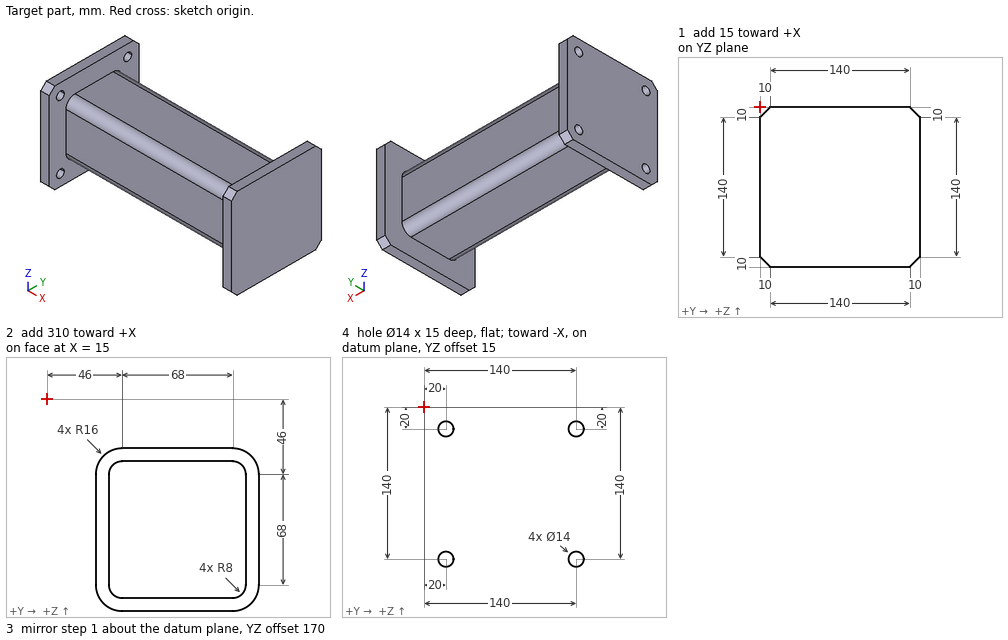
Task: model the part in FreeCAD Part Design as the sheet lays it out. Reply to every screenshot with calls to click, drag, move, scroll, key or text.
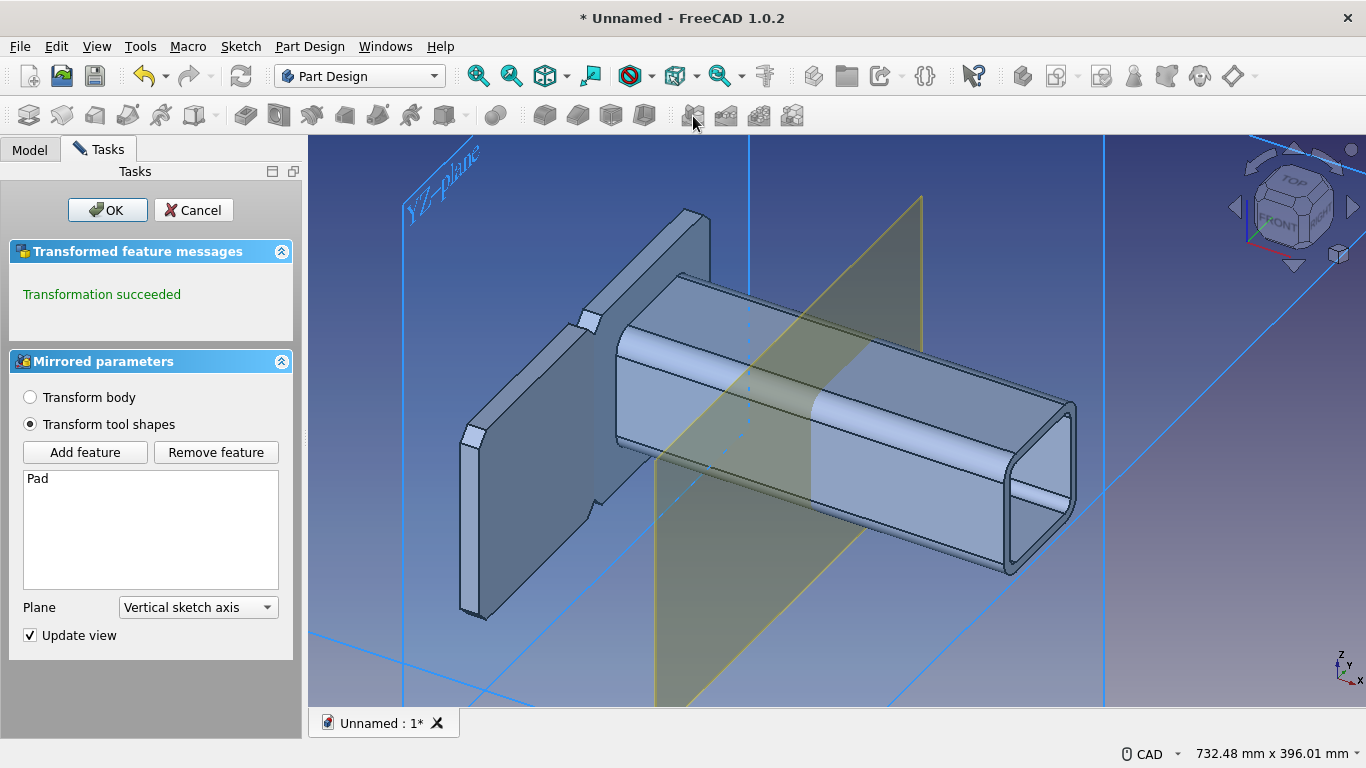
click(199, 608)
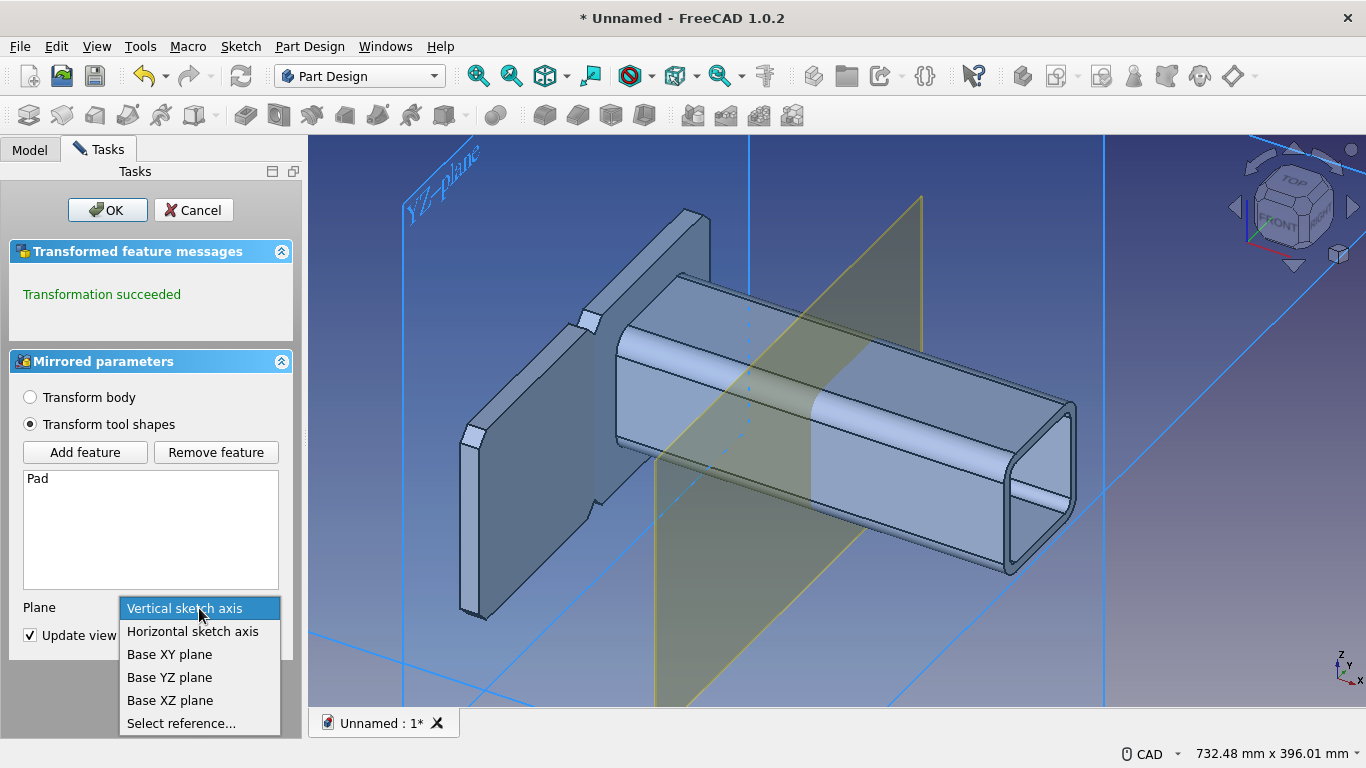
click(198, 724)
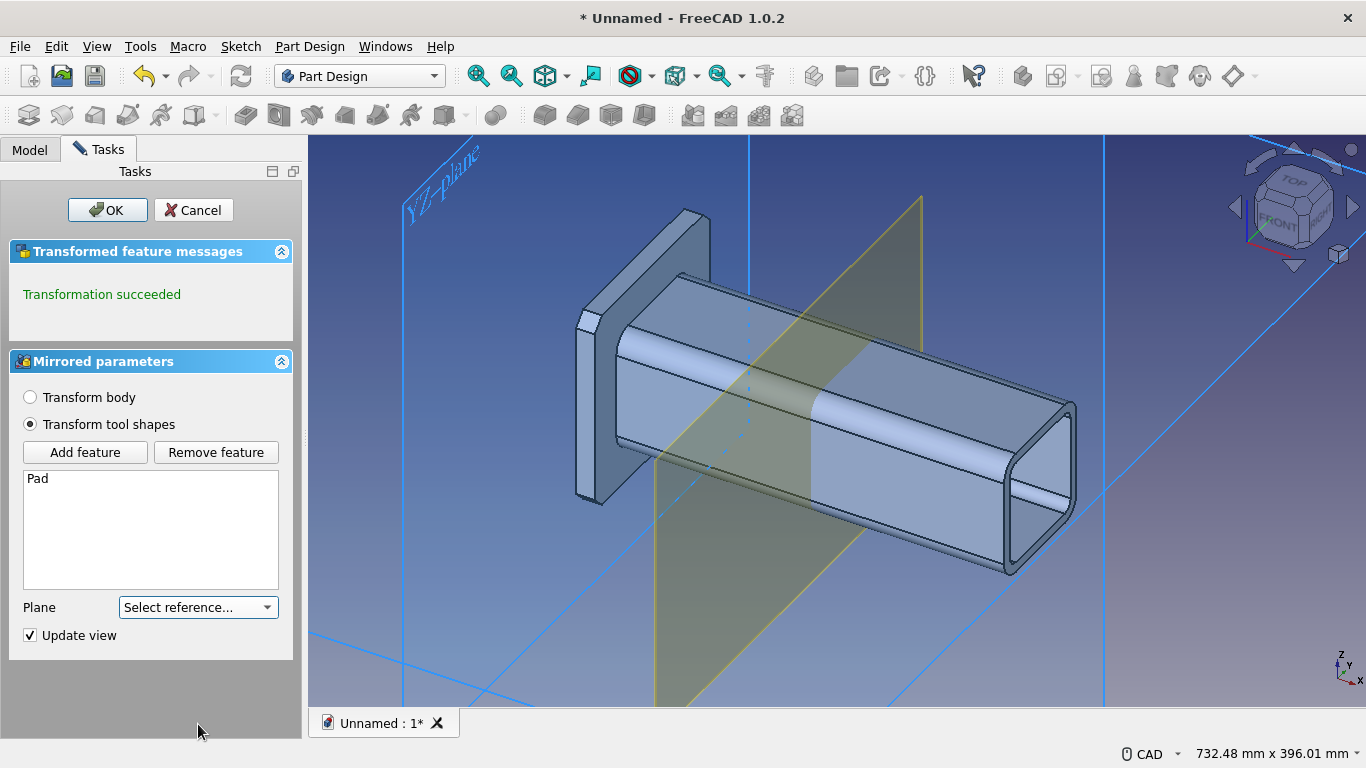
click(30, 149)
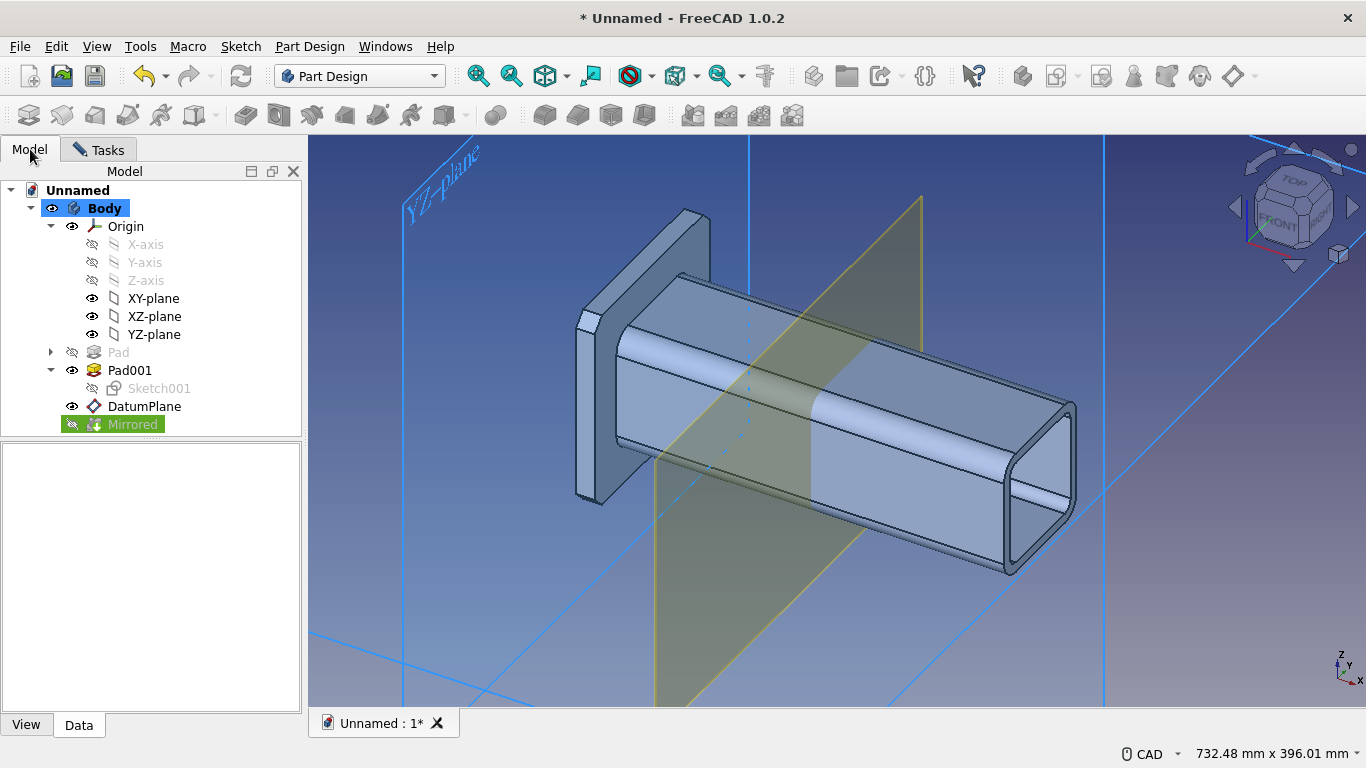
click(117, 406)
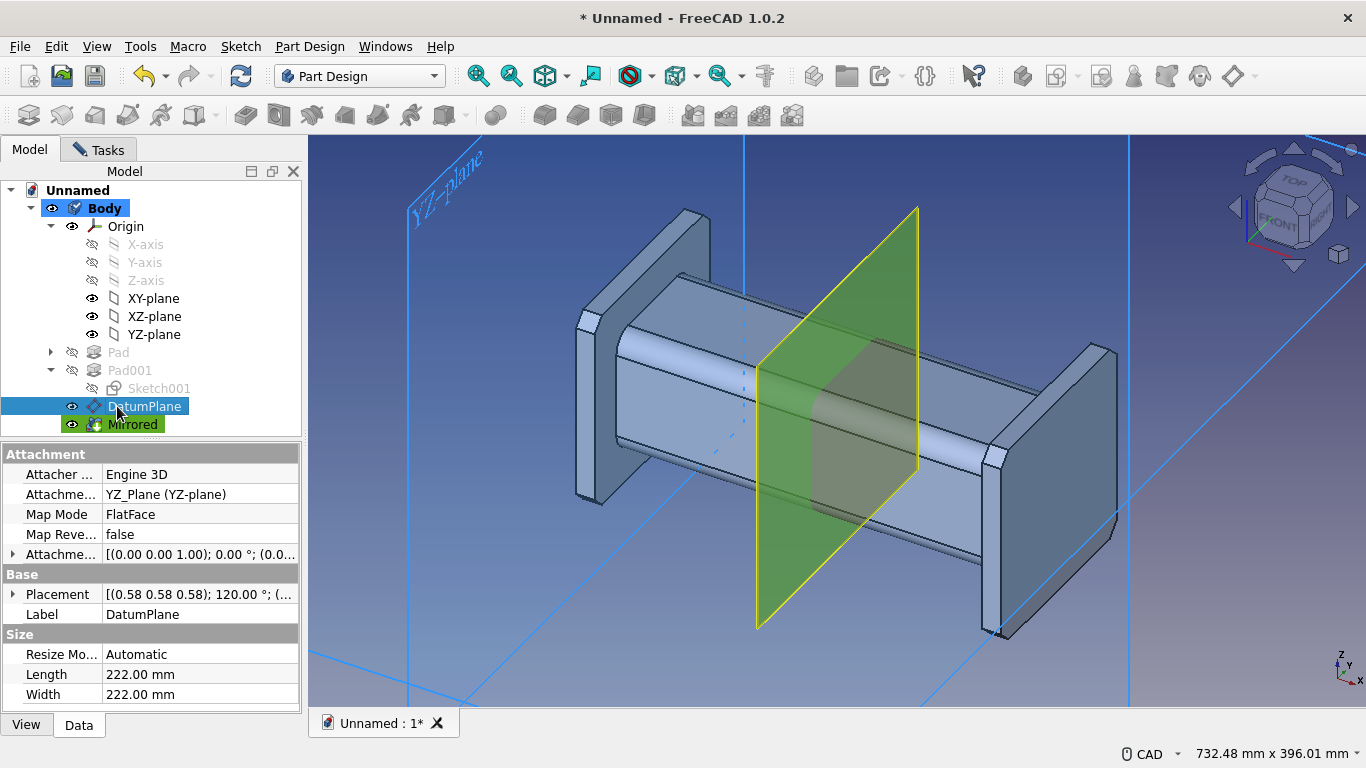
click(98, 149)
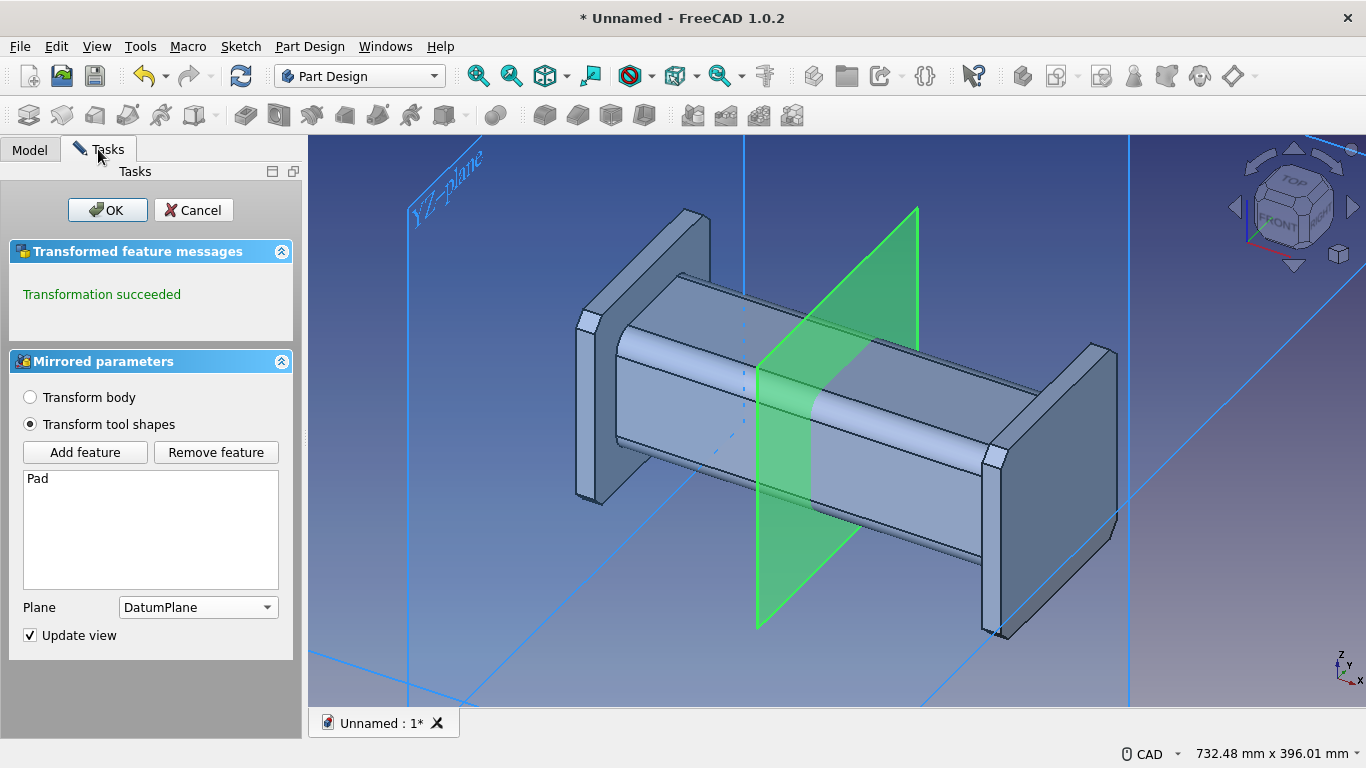
click(108, 210)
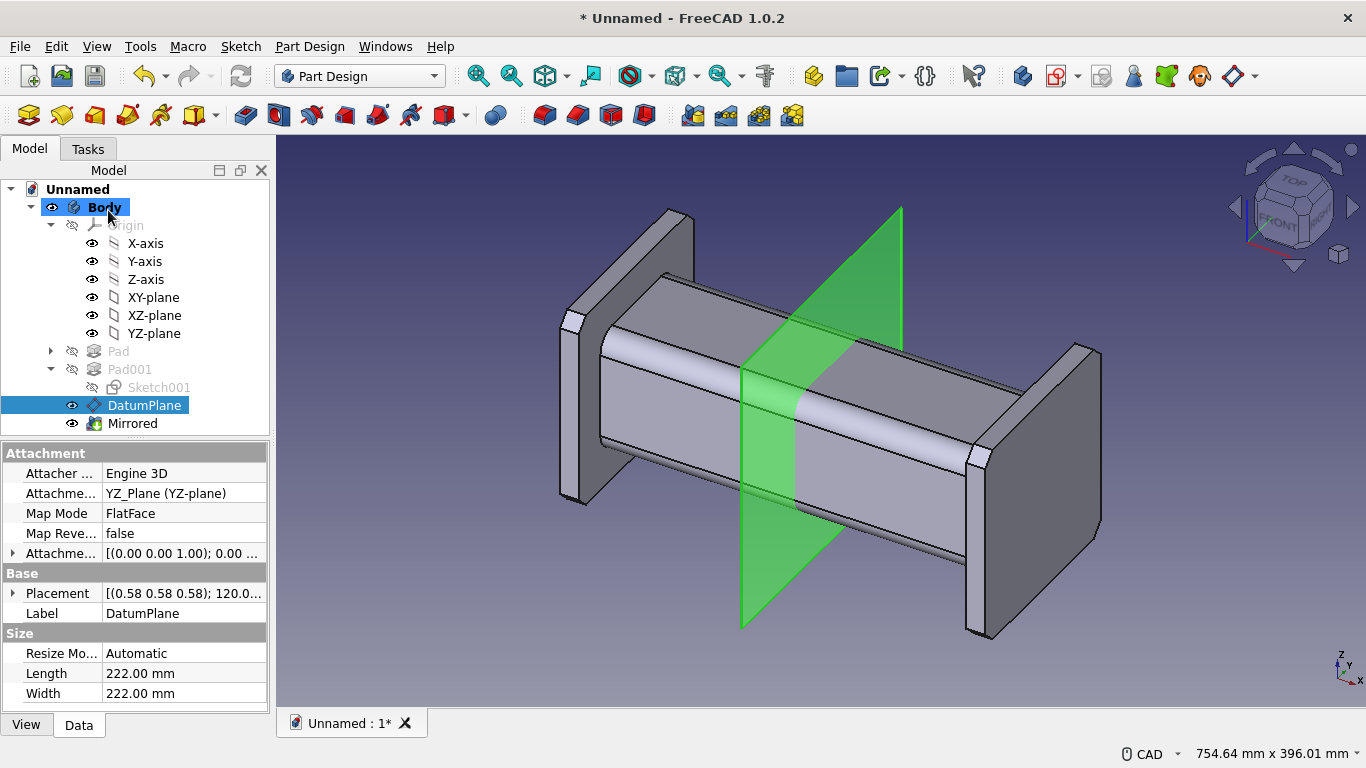
click(117, 405)
key(space)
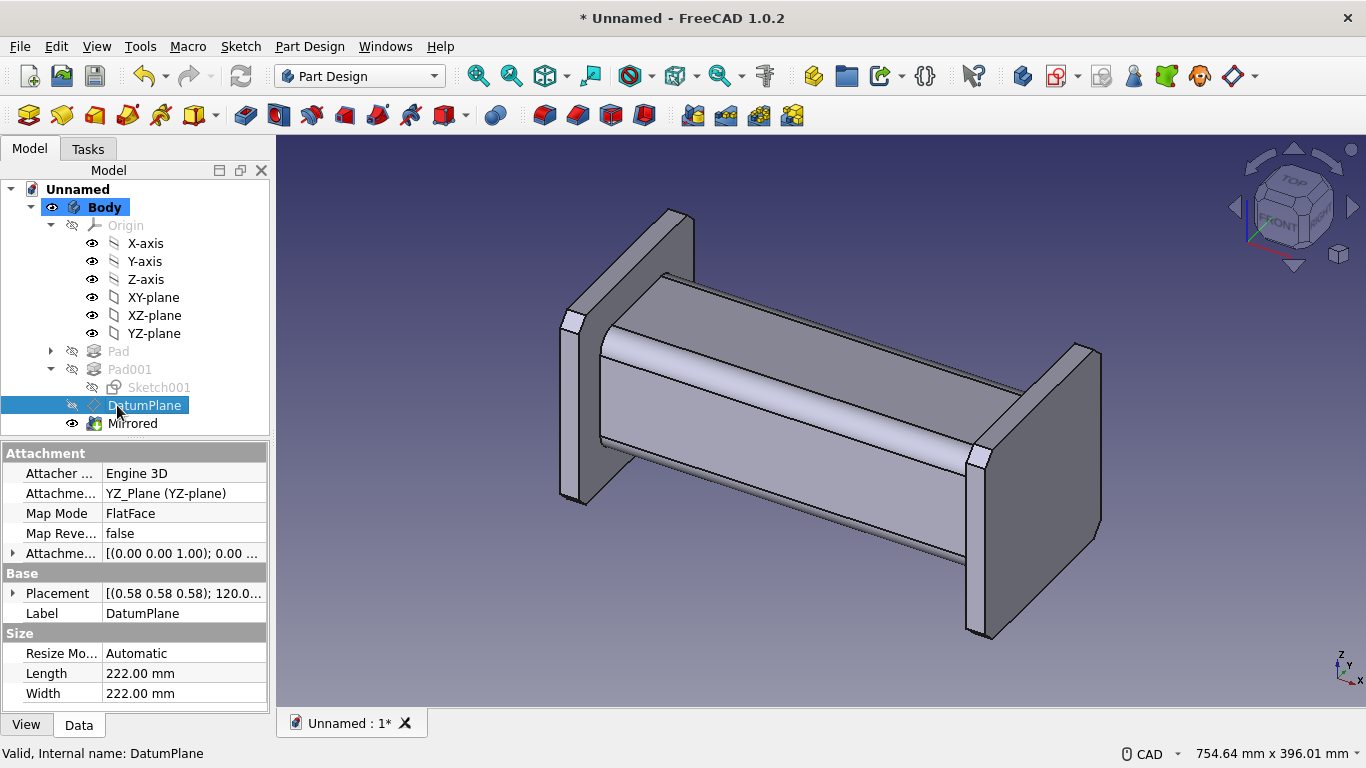
click(137, 333)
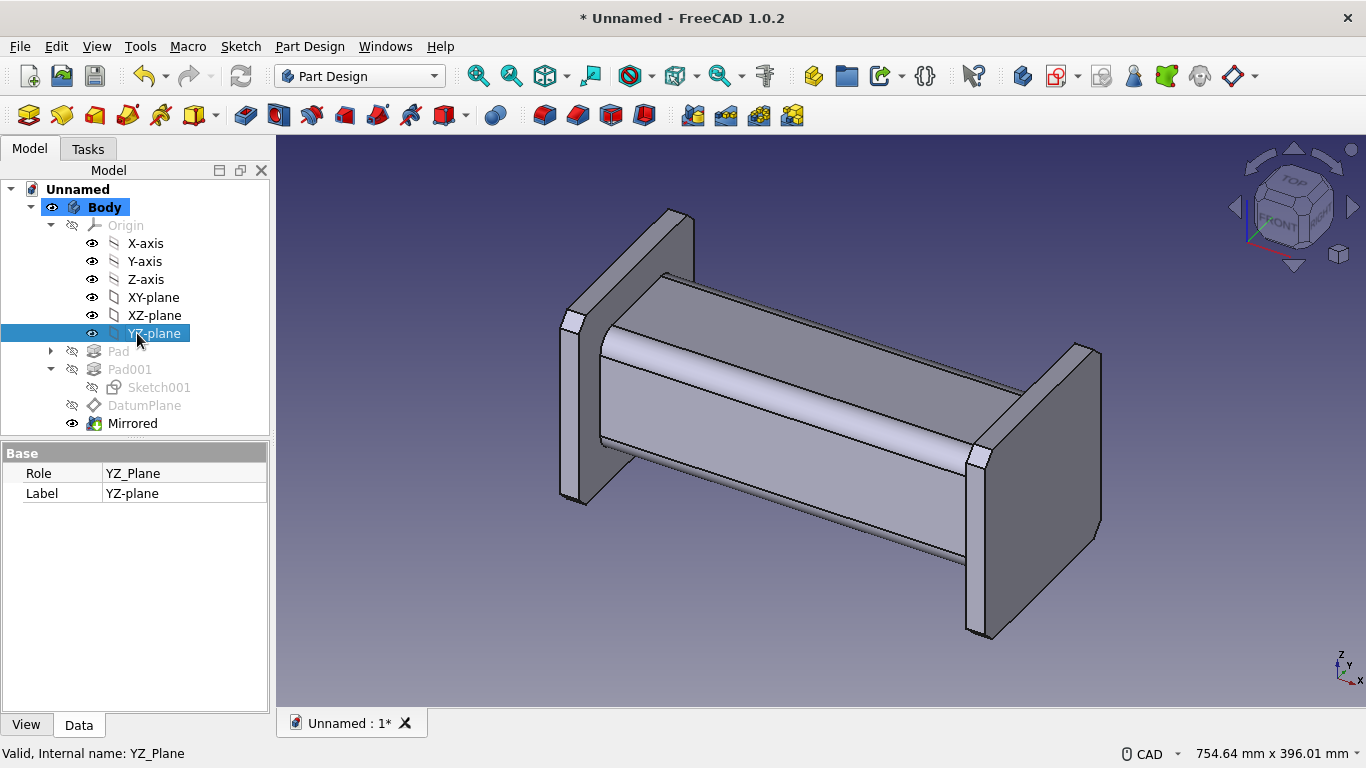
click(1232, 76)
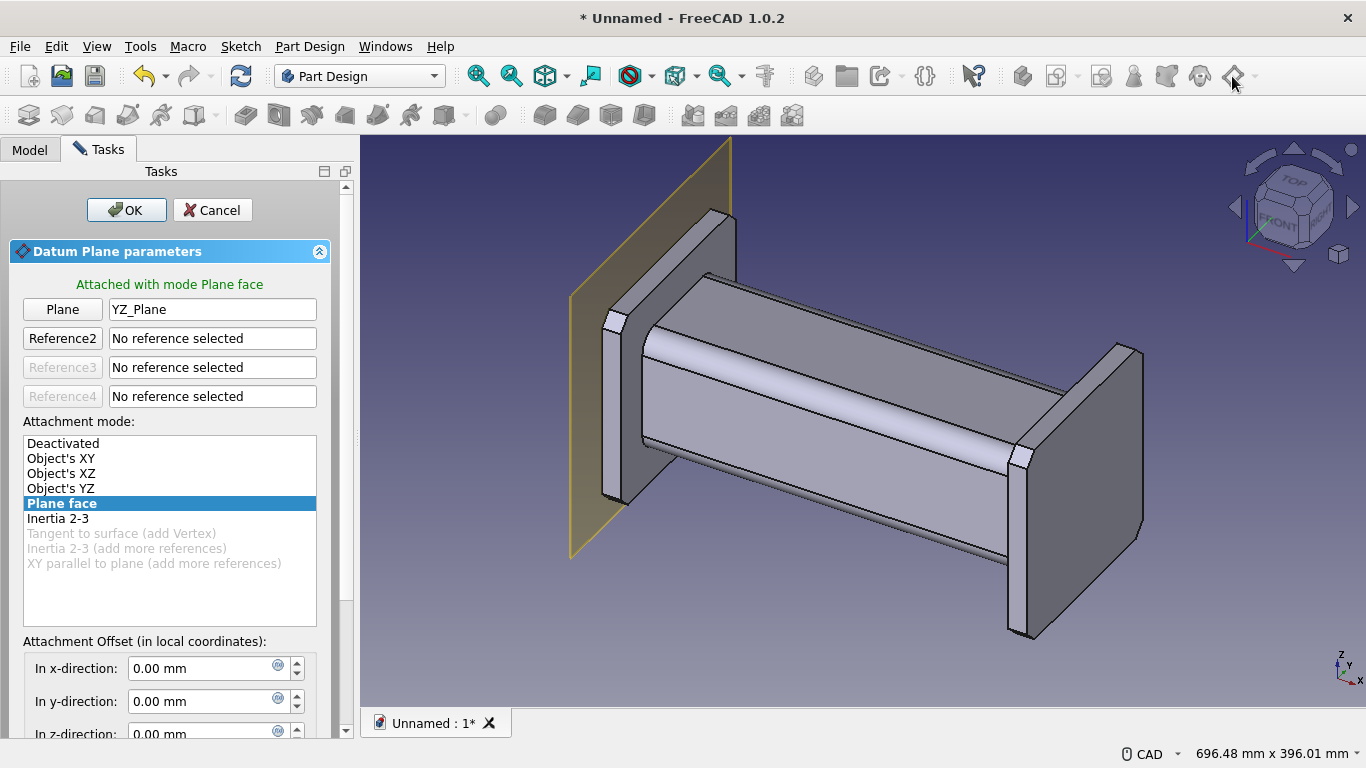
scroll(346, 460, down, 2)